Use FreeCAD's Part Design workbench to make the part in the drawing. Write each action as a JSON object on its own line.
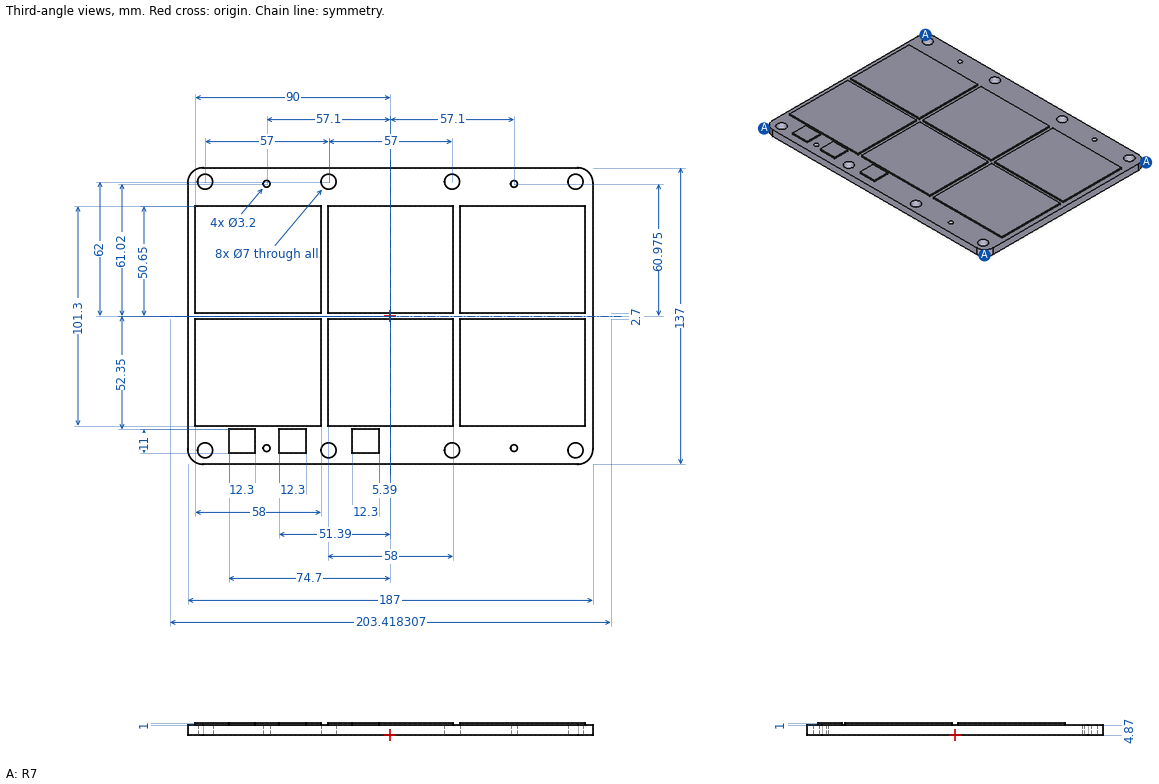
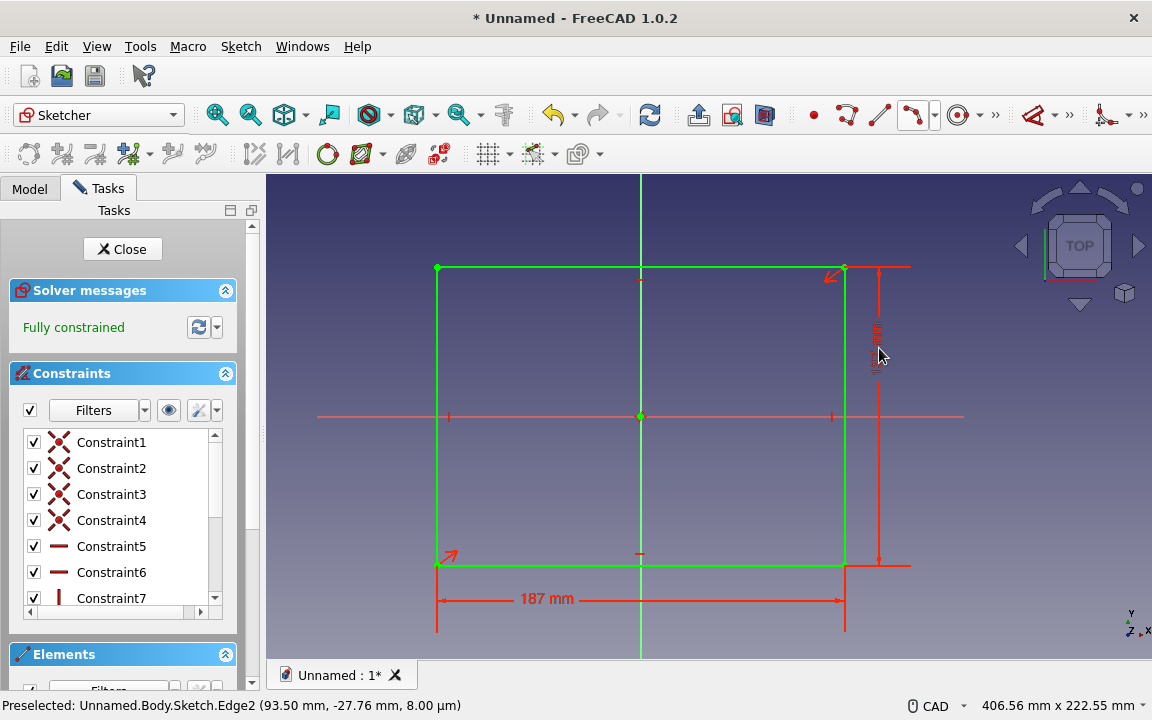
{"action": "left_click", "coordinate": [123, 249]}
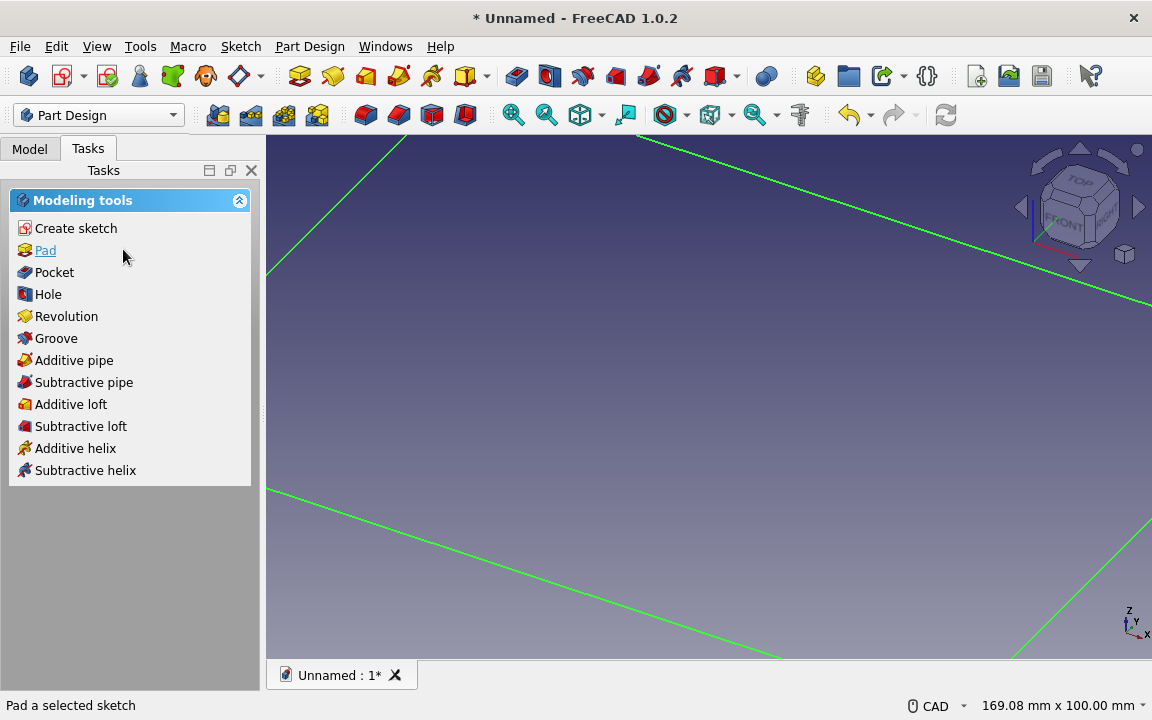
{"action": "left_click", "coordinate": [300, 76]}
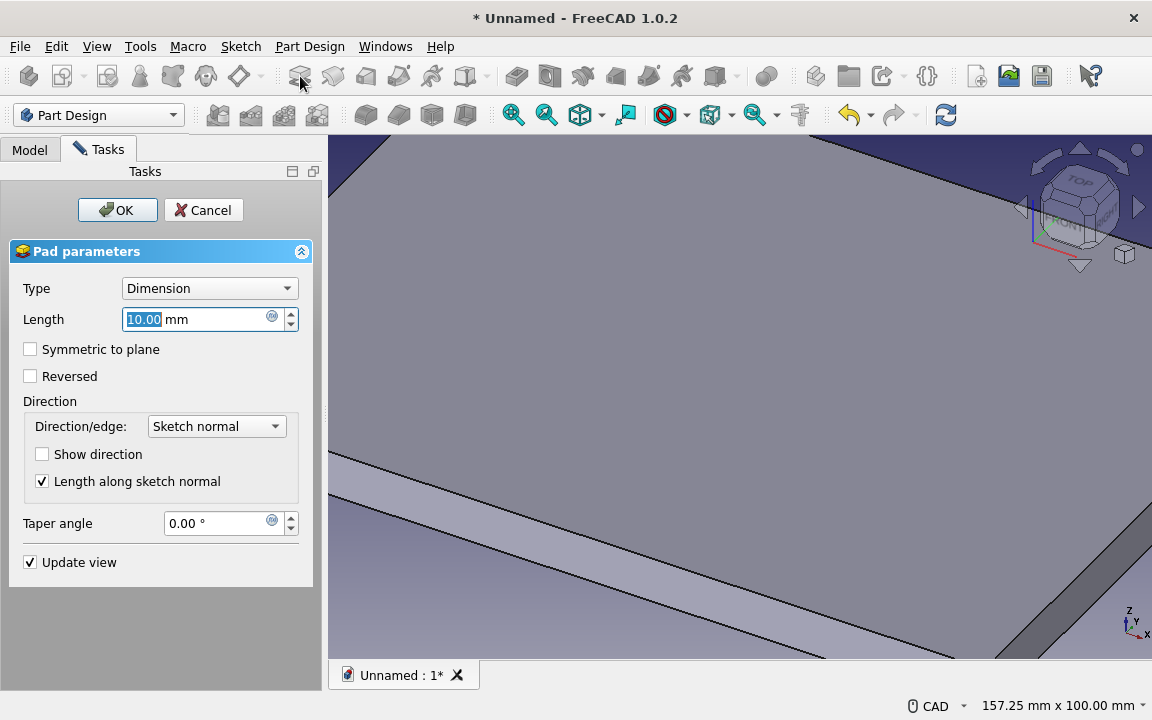
{"action": "type", "text": "4.87"}
{"action": "key", "text": "Tab"}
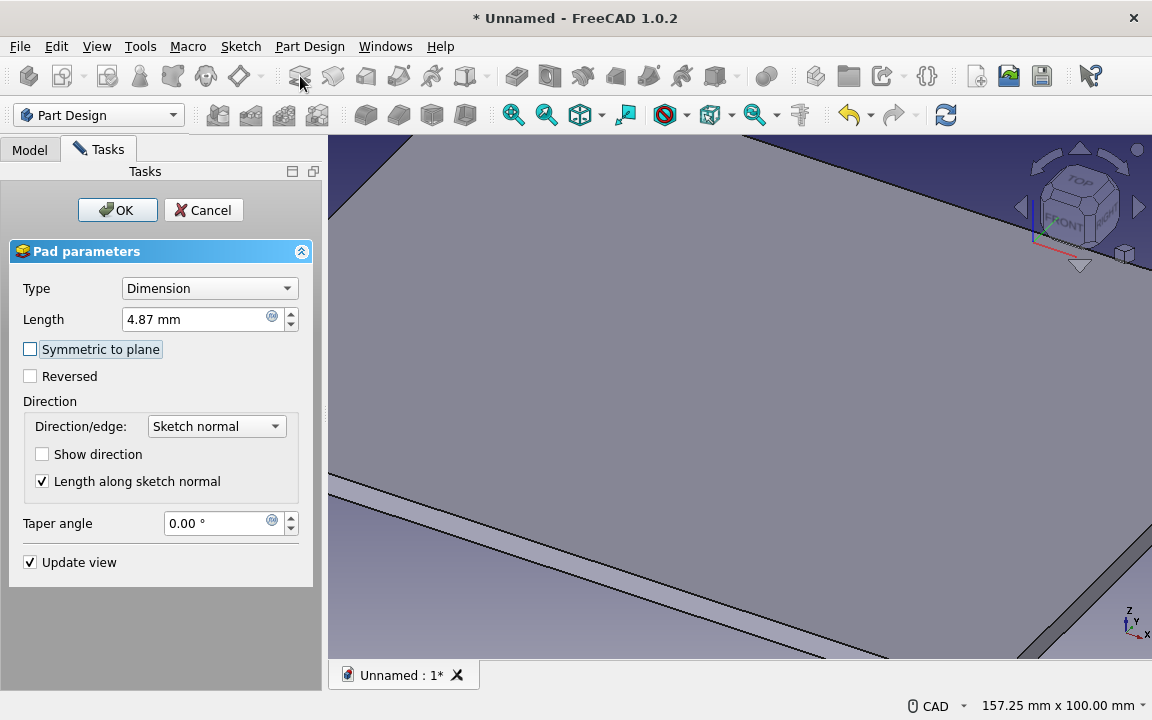
{"action": "left_click", "coordinate": [118, 210]}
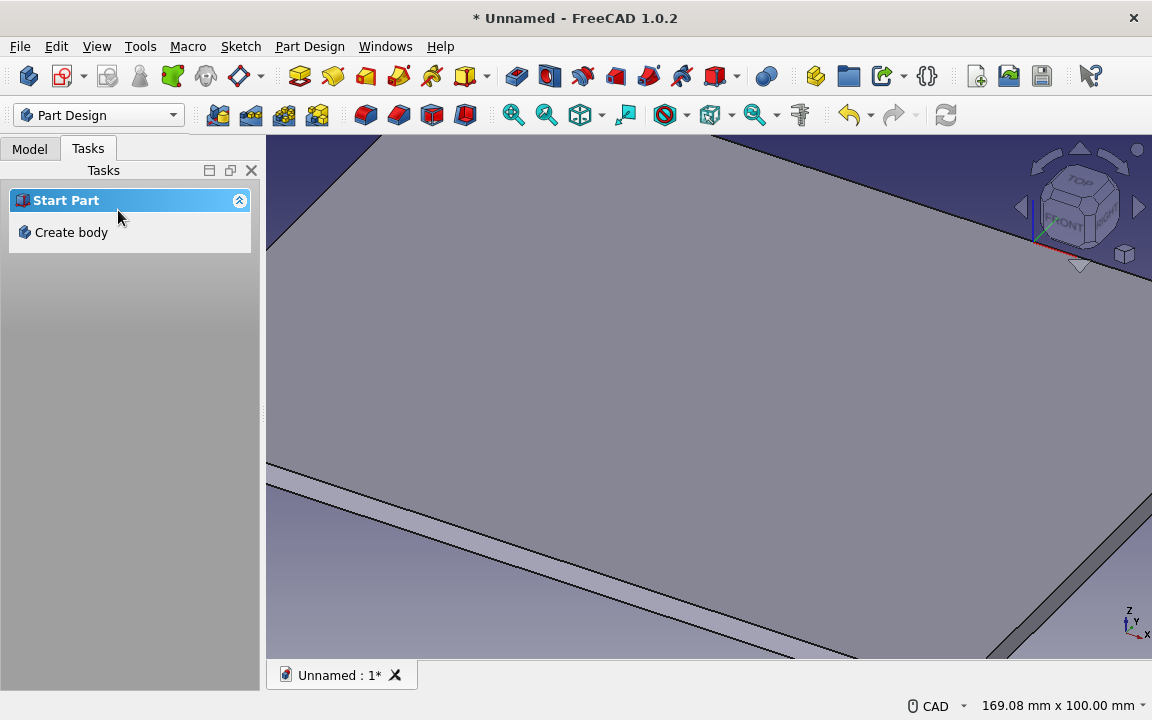
{"action": "key", "text": "v f"}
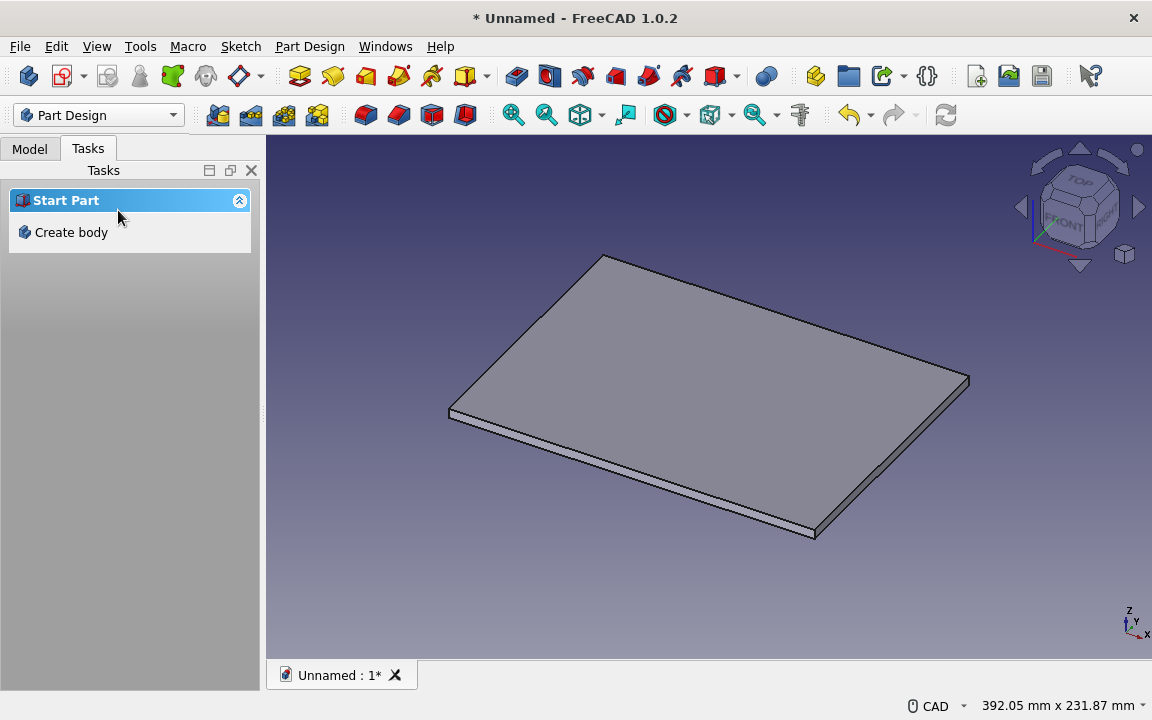
{"action": "left_click", "coordinate": [709, 391]}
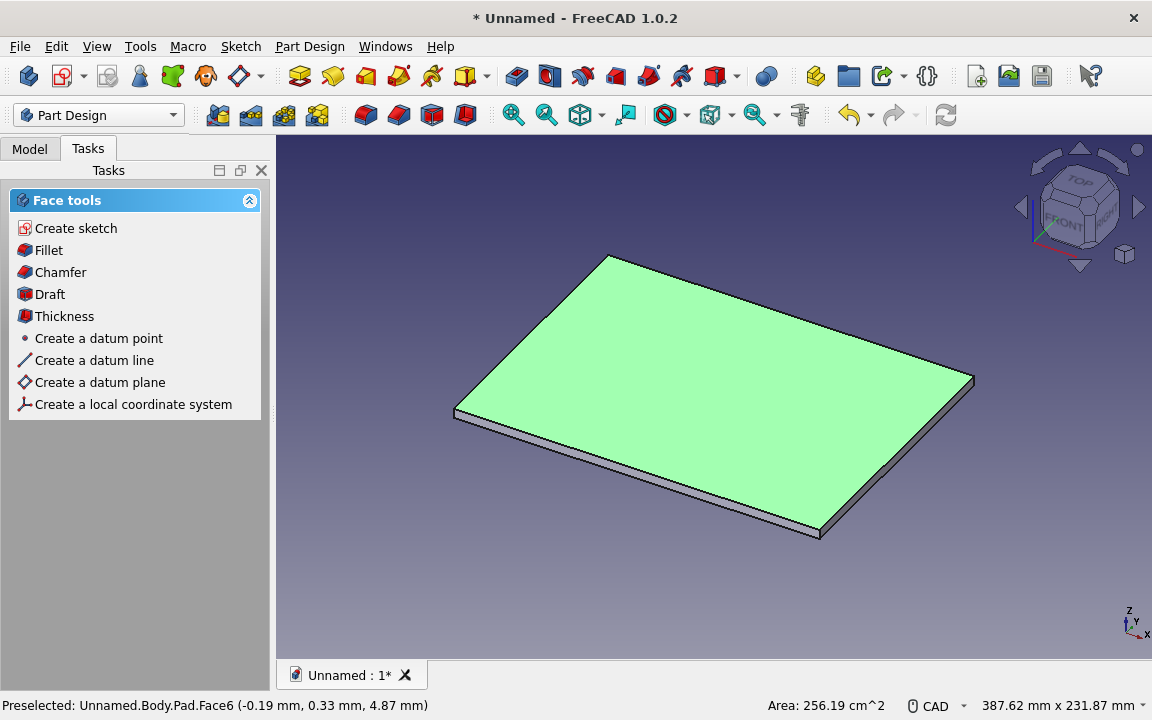
{"action": "left_click", "coordinate": [62, 76]}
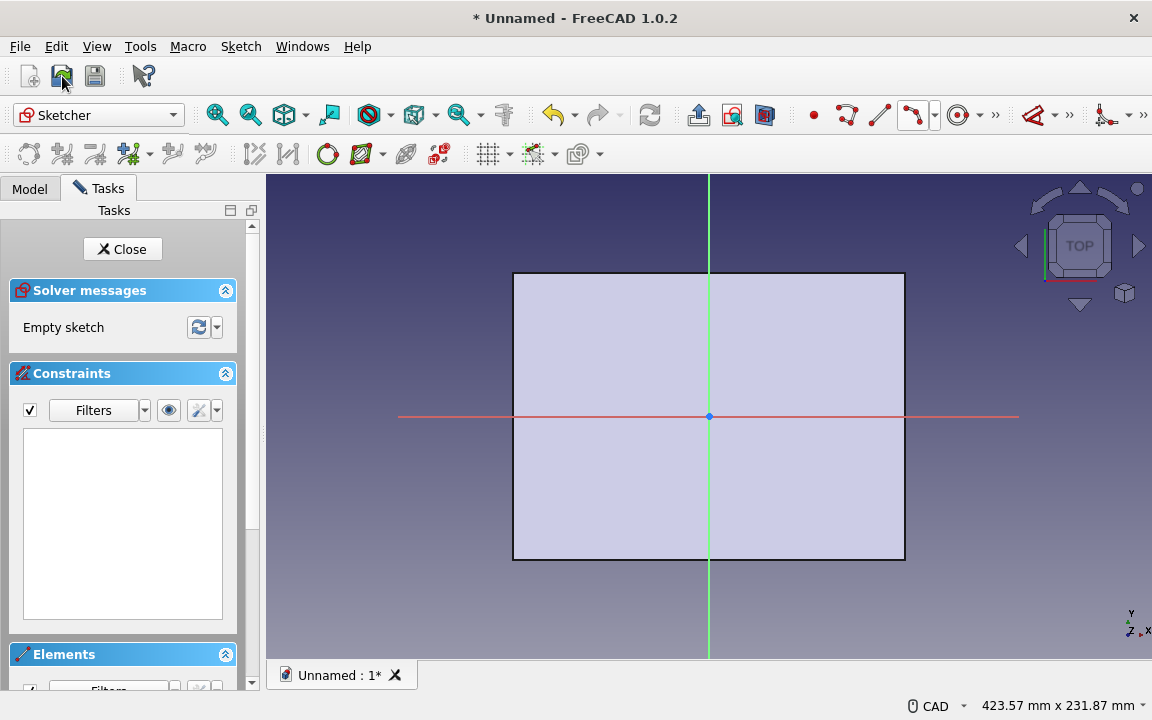
{"action": "key", "text": "g c"}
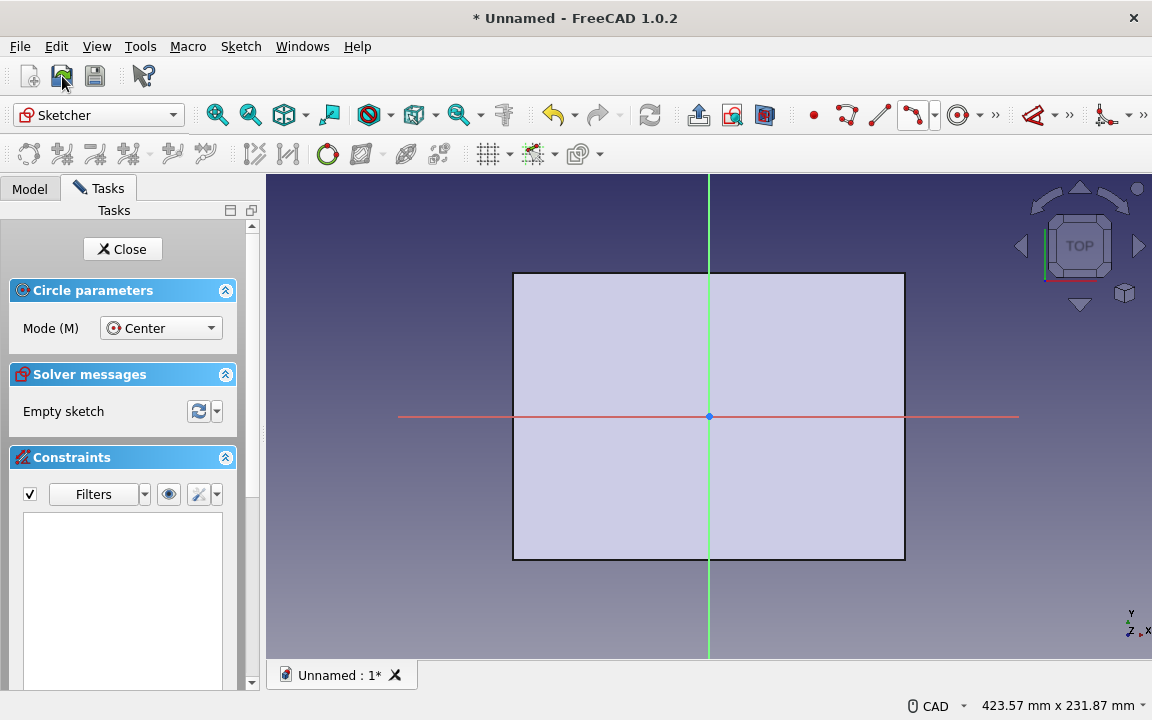
{"action": "scroll", "coordinate": [649, 287], "scroll_direction": "up", "scroll_amount": 6}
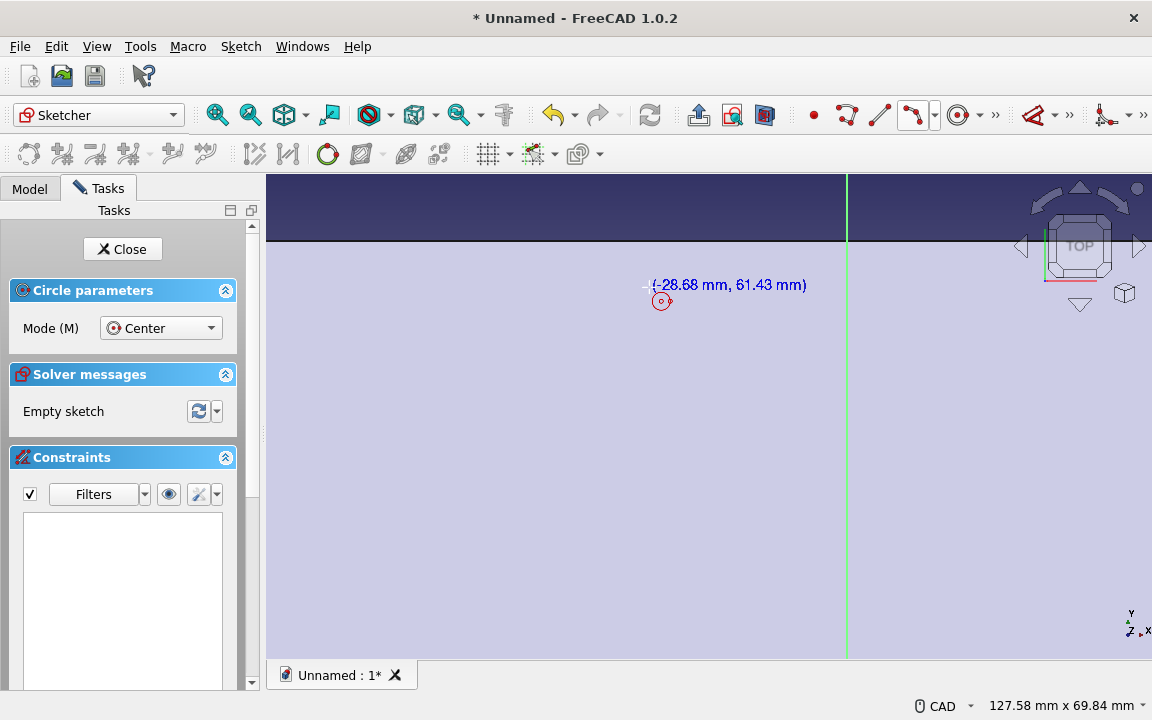
{"action": "left_click", "coordinate": [649, 286]}
{"action": "left_click", "coordinate": [666, 269]}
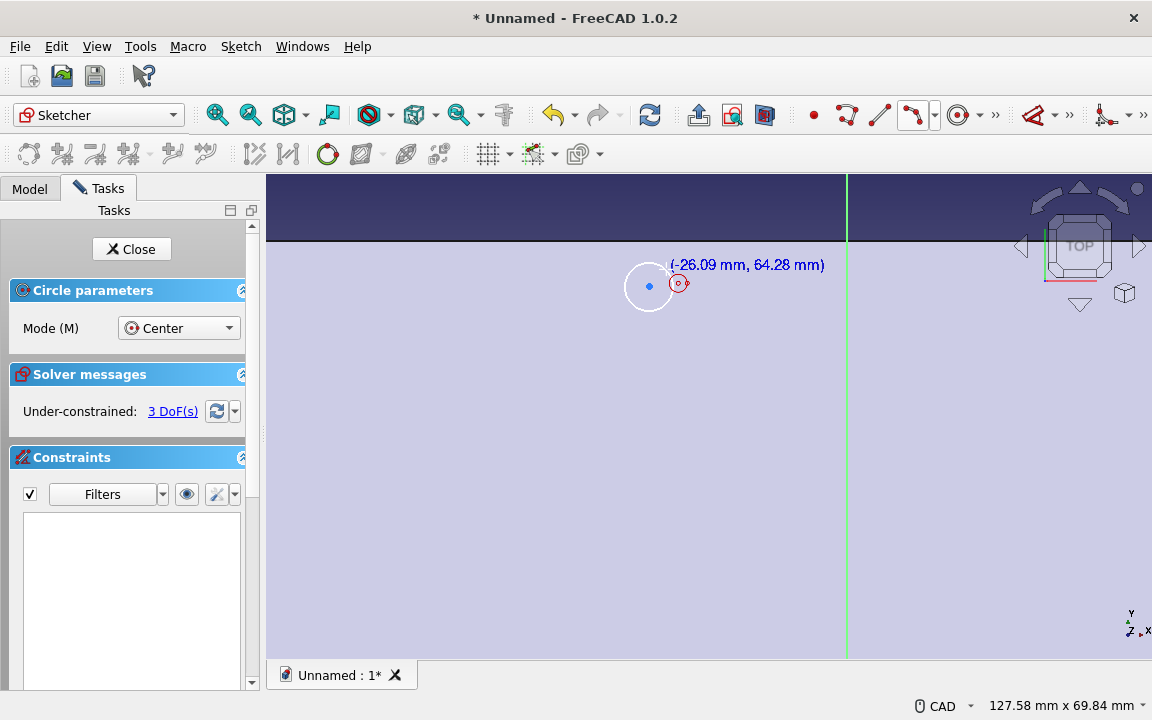
{"action": "scroll", "coordinate": [551, 287], "scroll_direction": "down", "scroll_amount": 6}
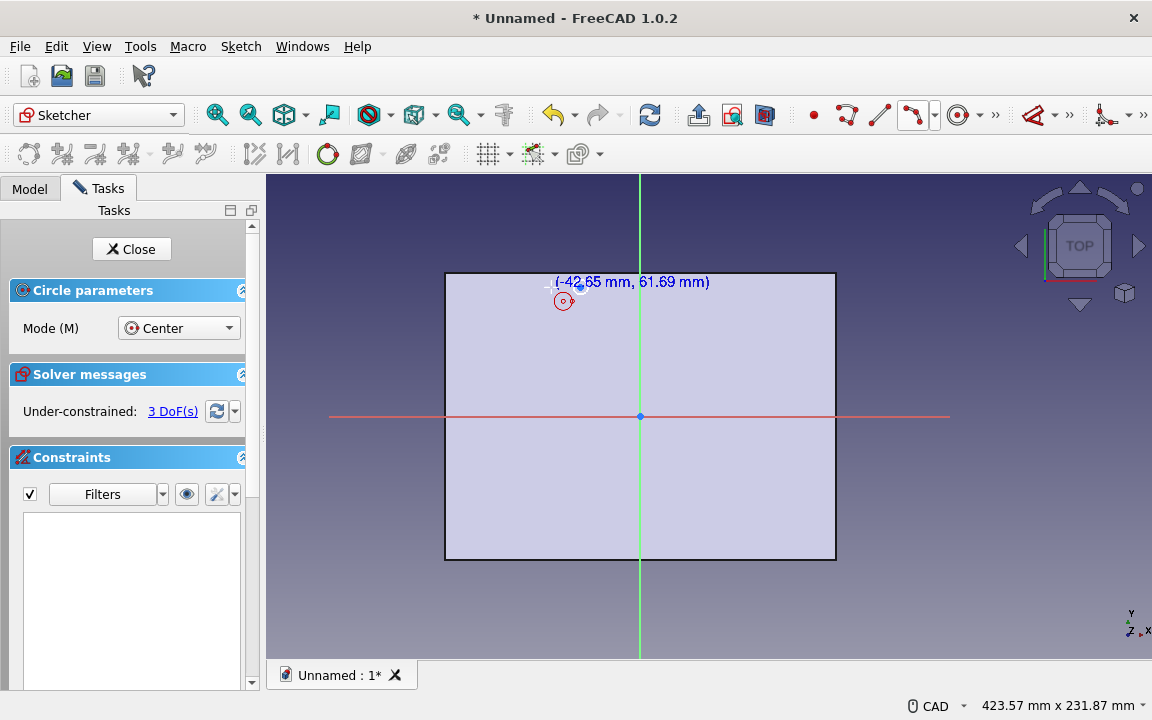
{"action": "scroll", "coordinate": [462, 287], "scroll_direction": "up", "scroll_amount": 6}